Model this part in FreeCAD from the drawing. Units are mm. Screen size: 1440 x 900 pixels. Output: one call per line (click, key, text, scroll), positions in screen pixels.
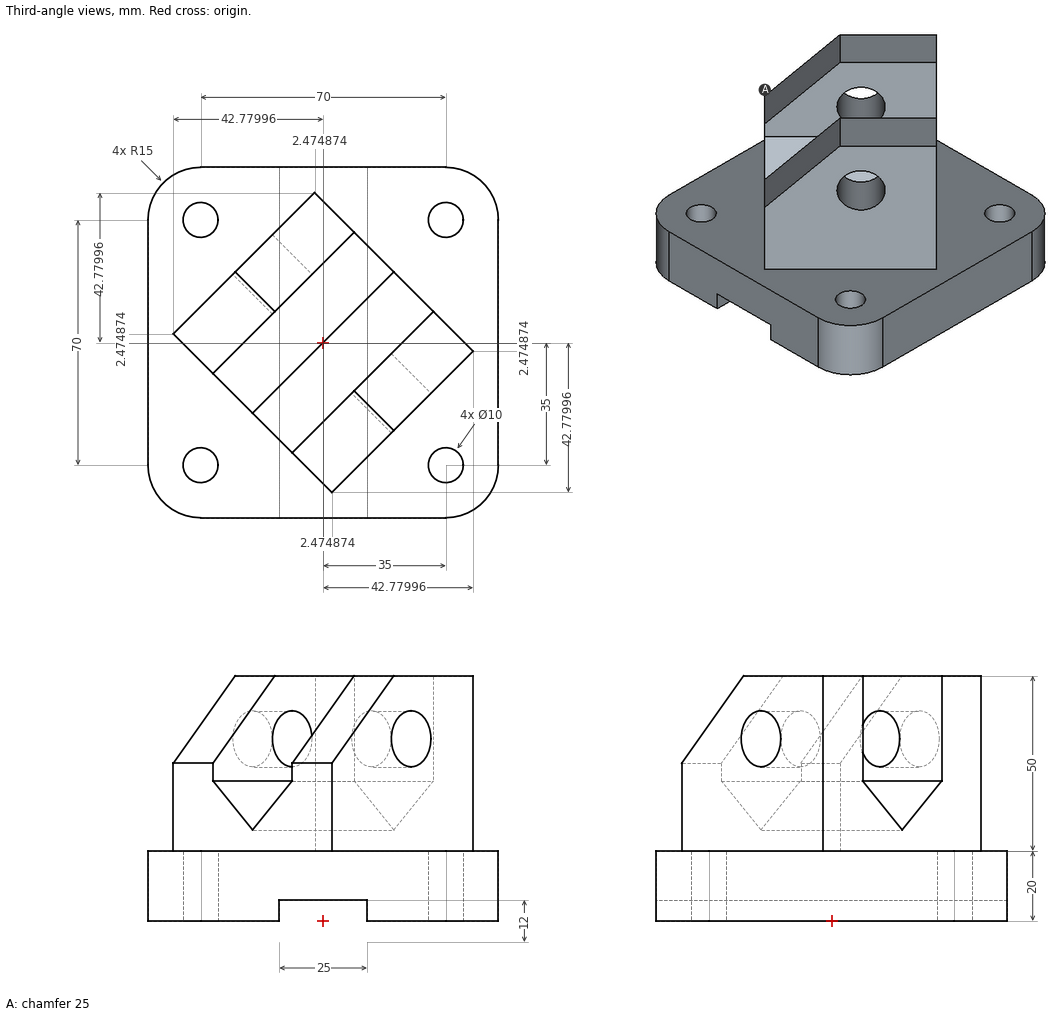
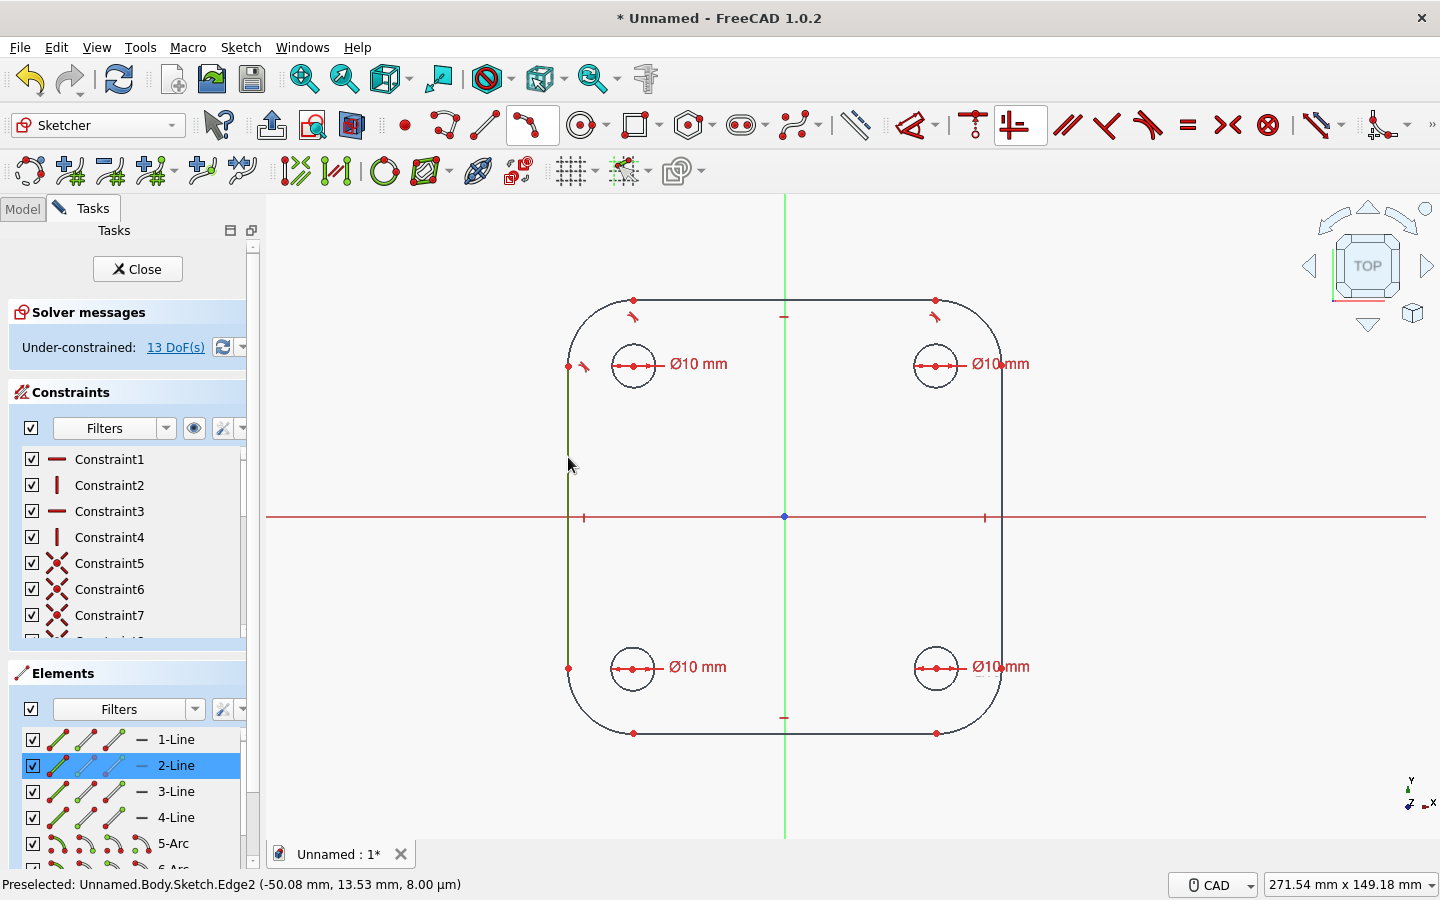
click(575, 699)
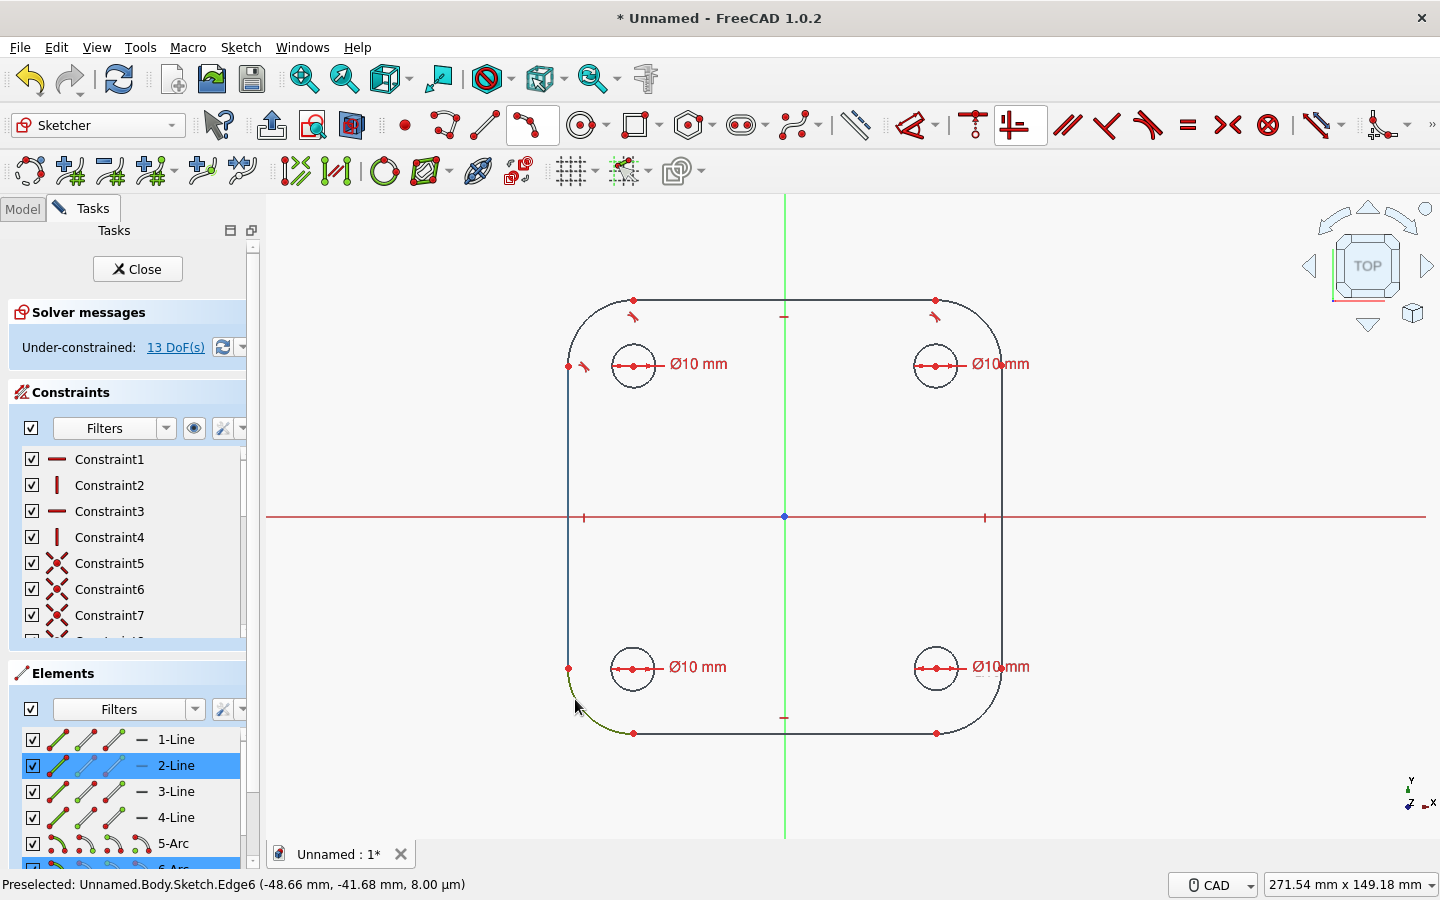
key(t)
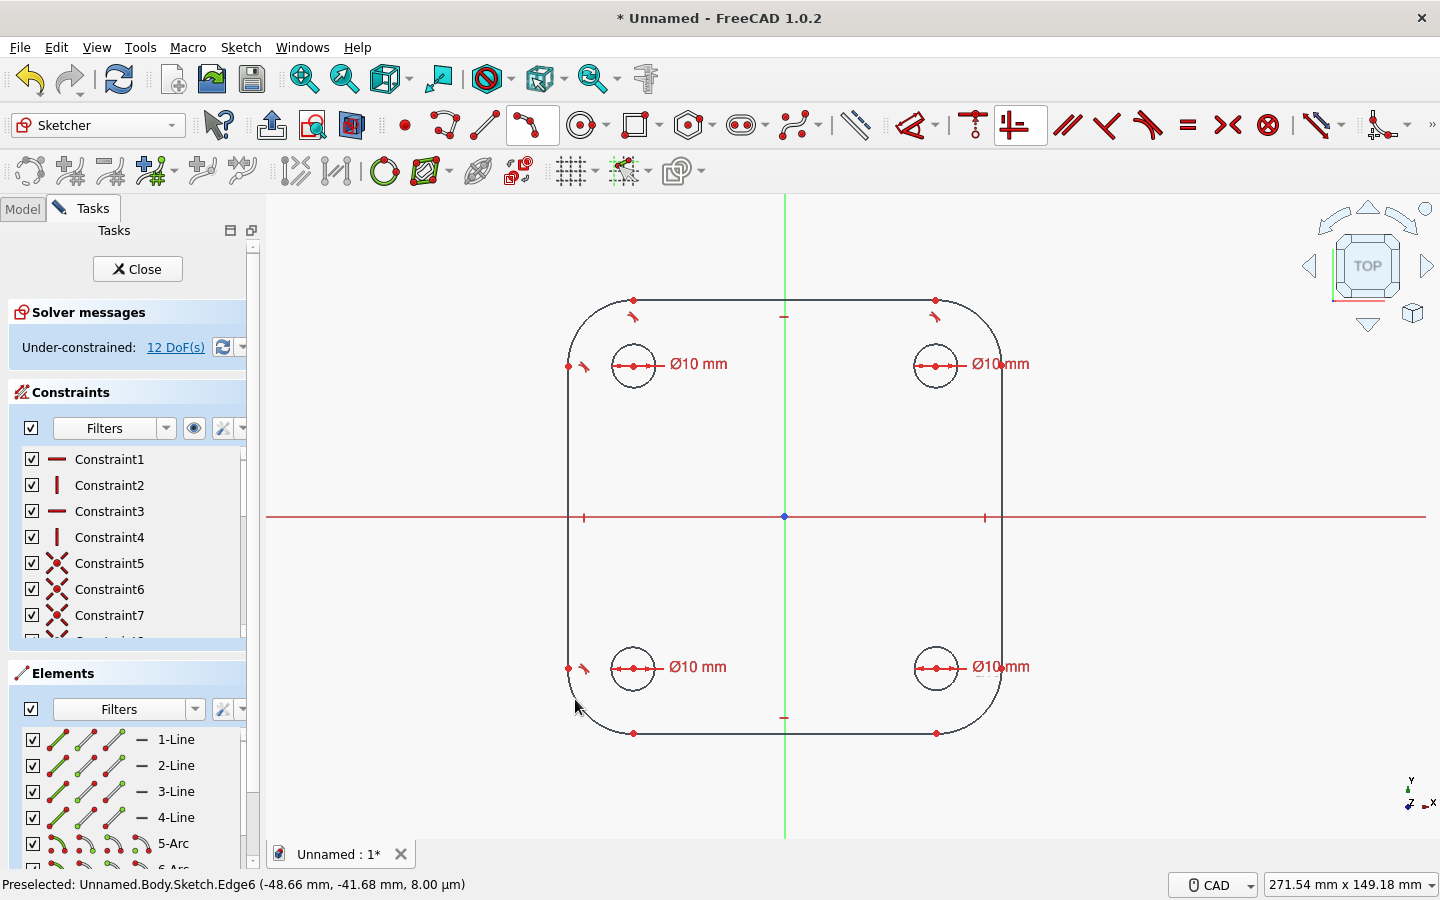
click(724, 734)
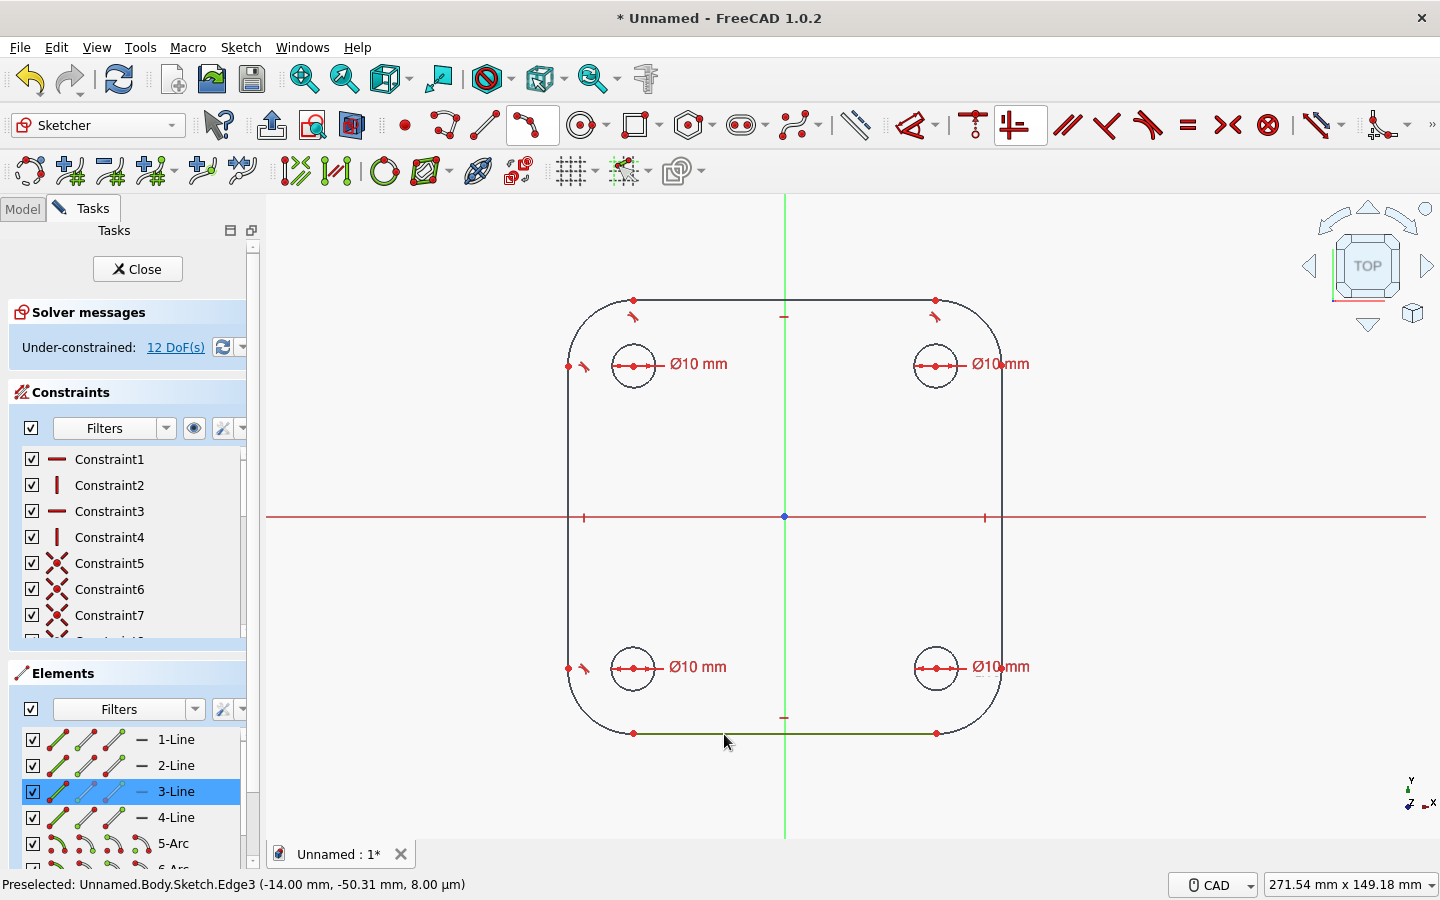
click(575, 699)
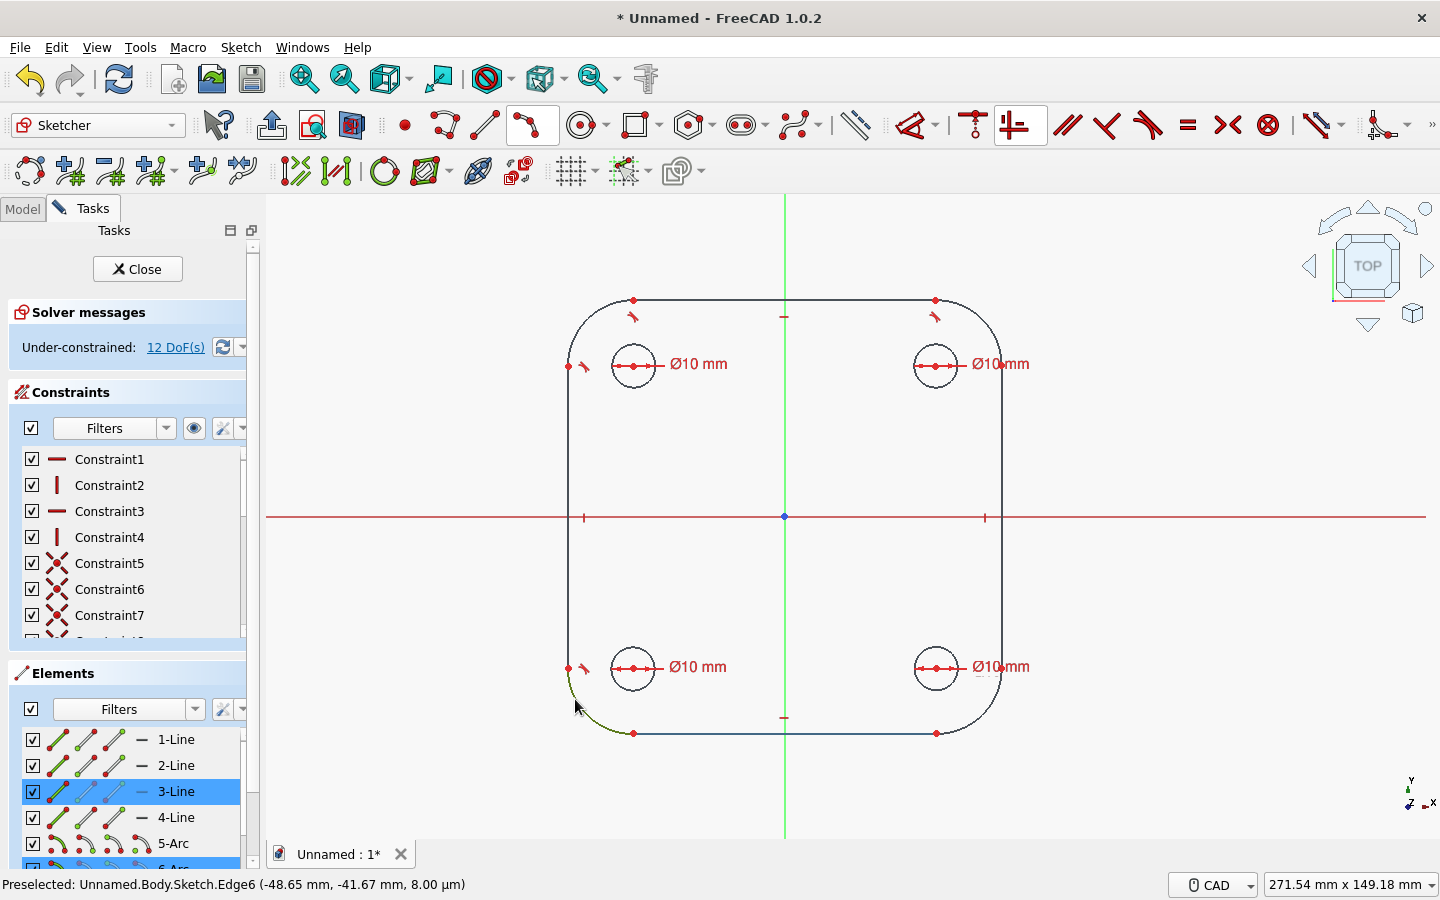
key(t)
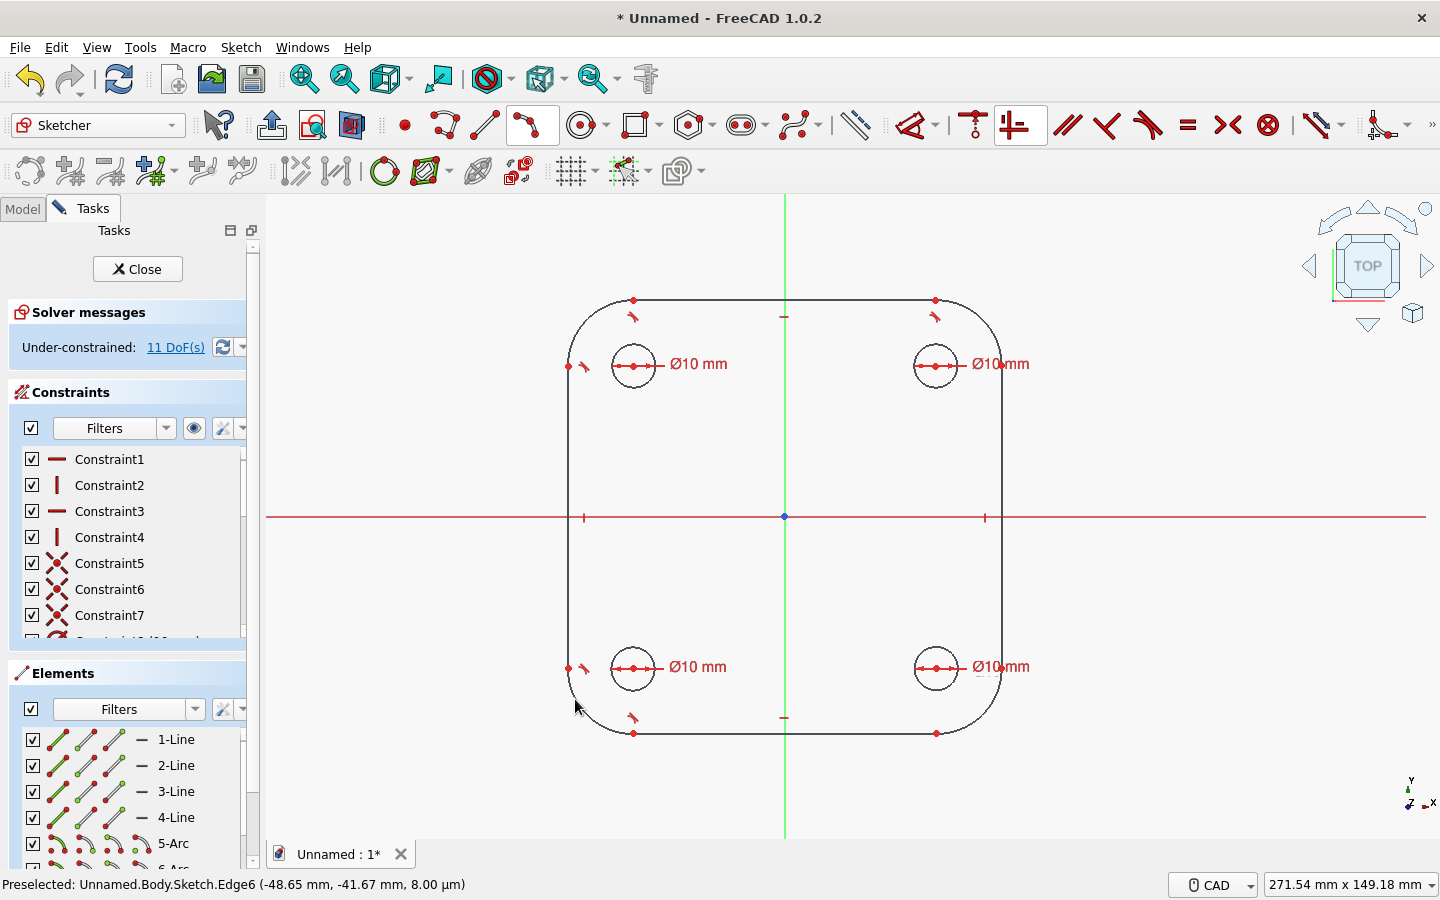
click(724, 734)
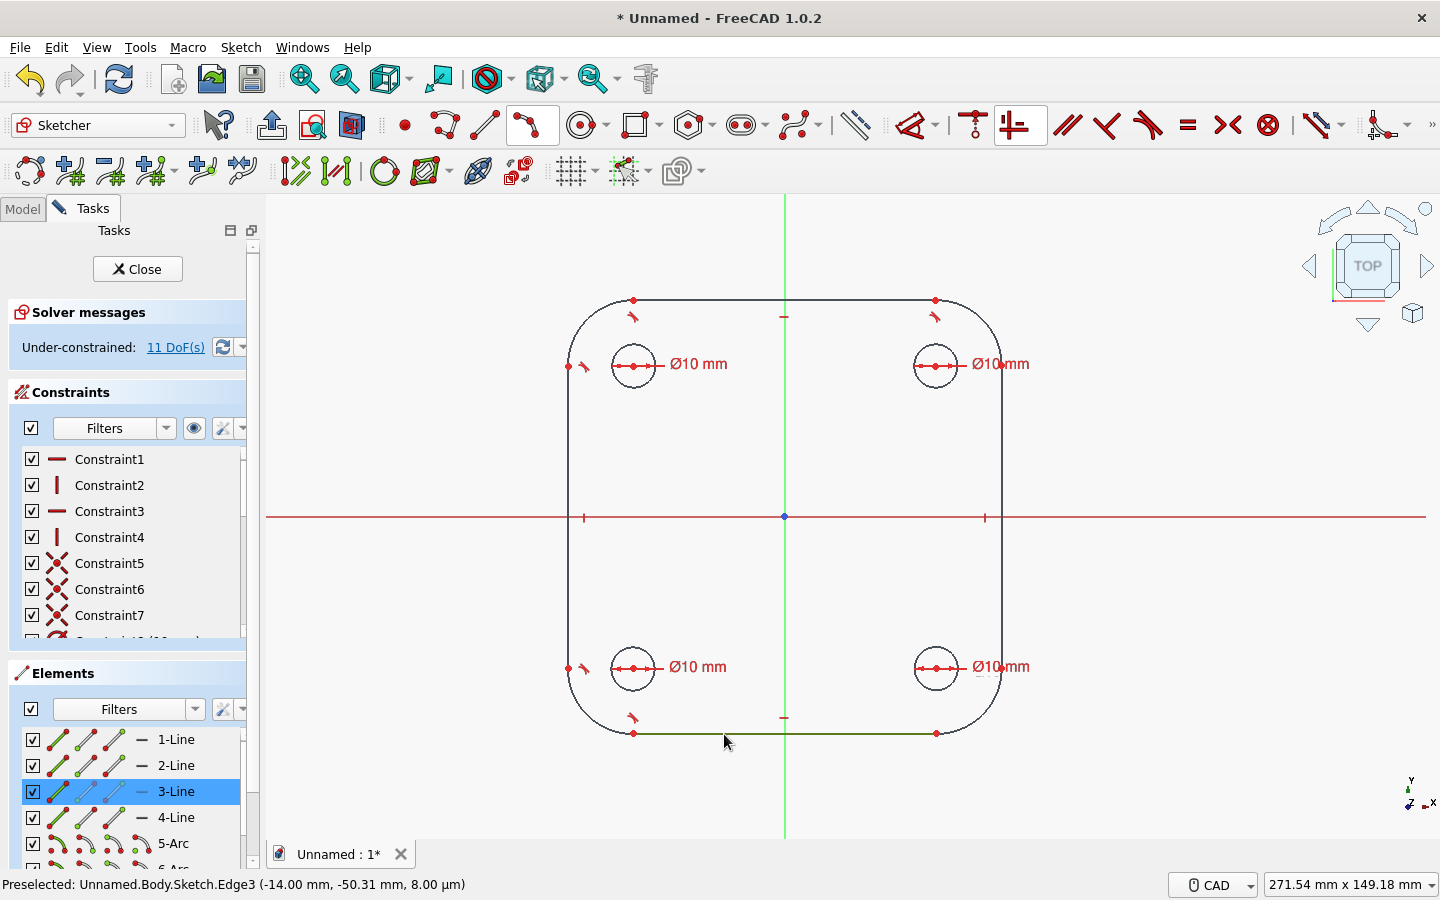
click(966, 727)